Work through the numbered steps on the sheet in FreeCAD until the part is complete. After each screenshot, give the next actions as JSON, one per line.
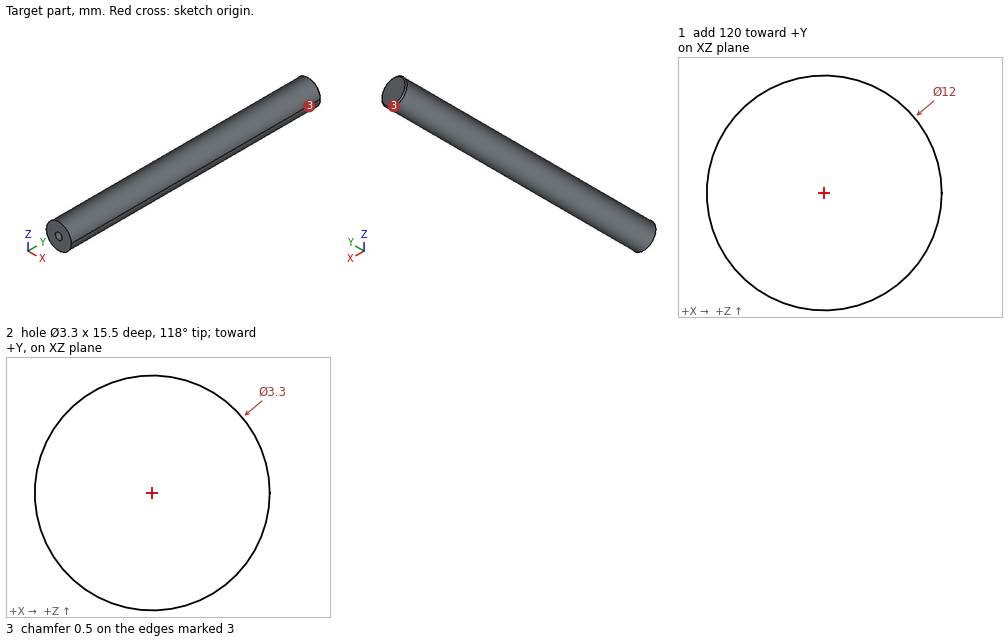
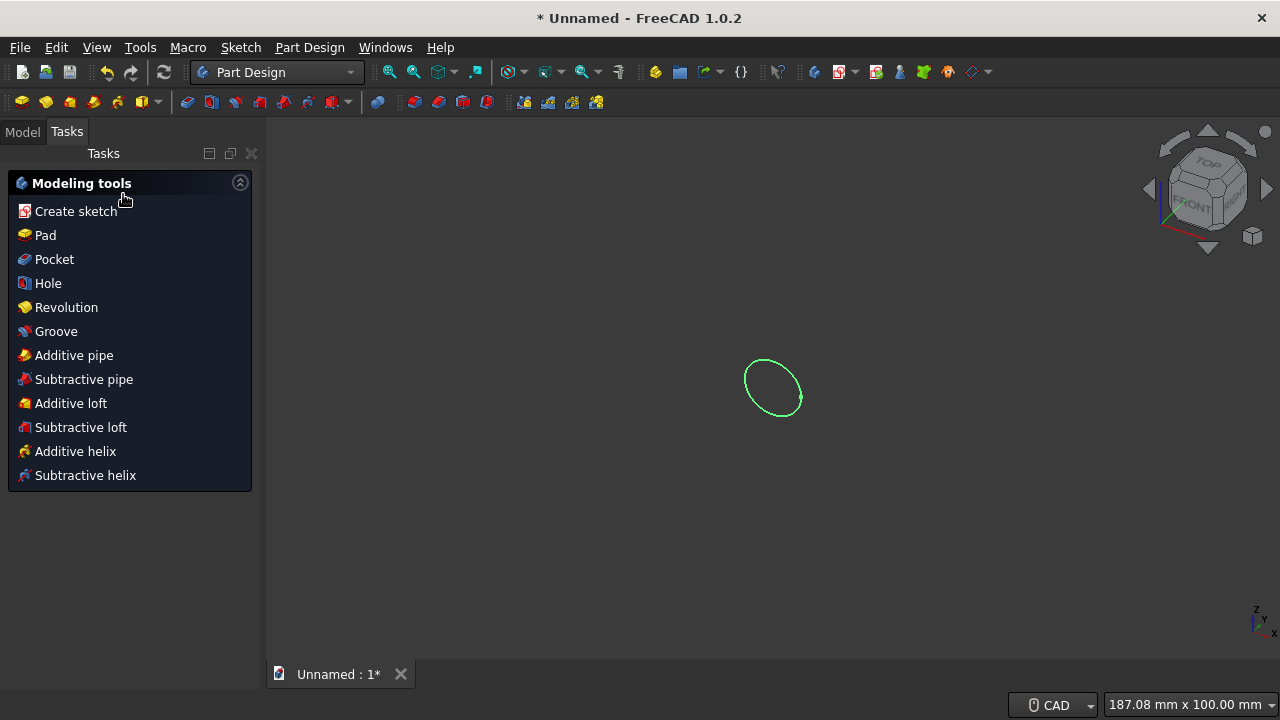
{"action": "left_click", "coordinate": [22, 102]}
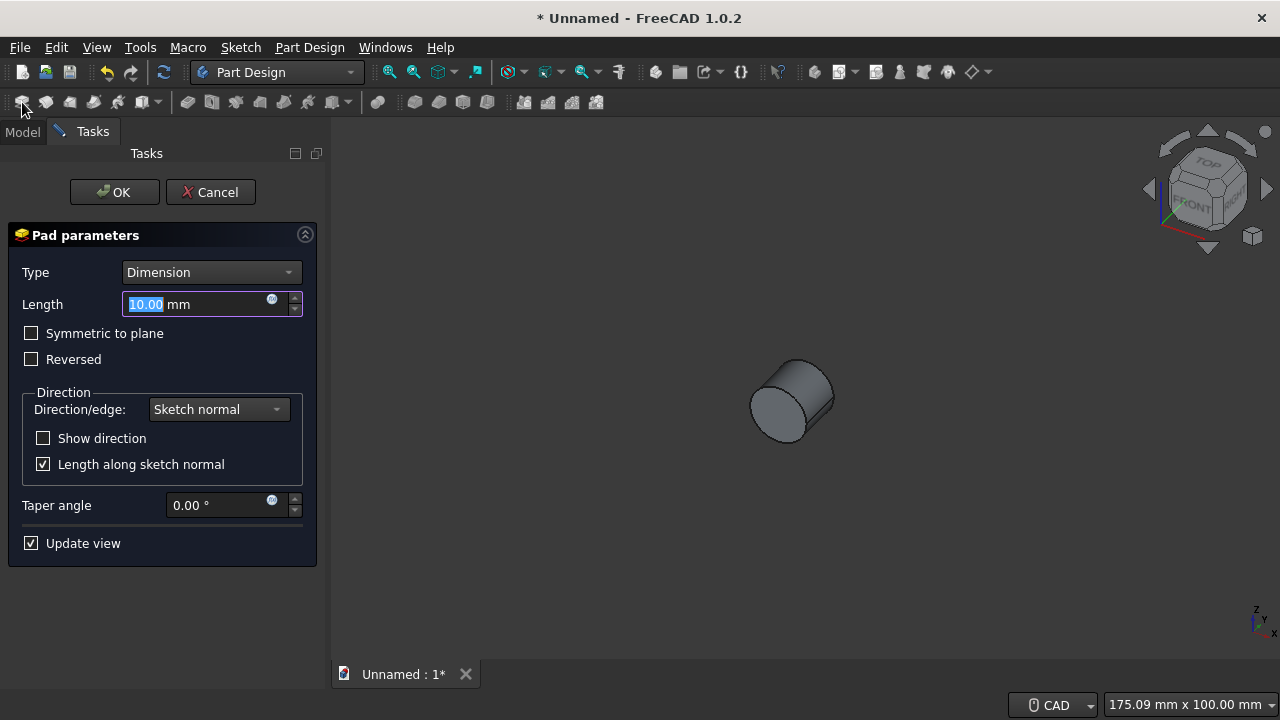
{"action": "type", "text": "120"}
{"action": "key", "text": "Tab"}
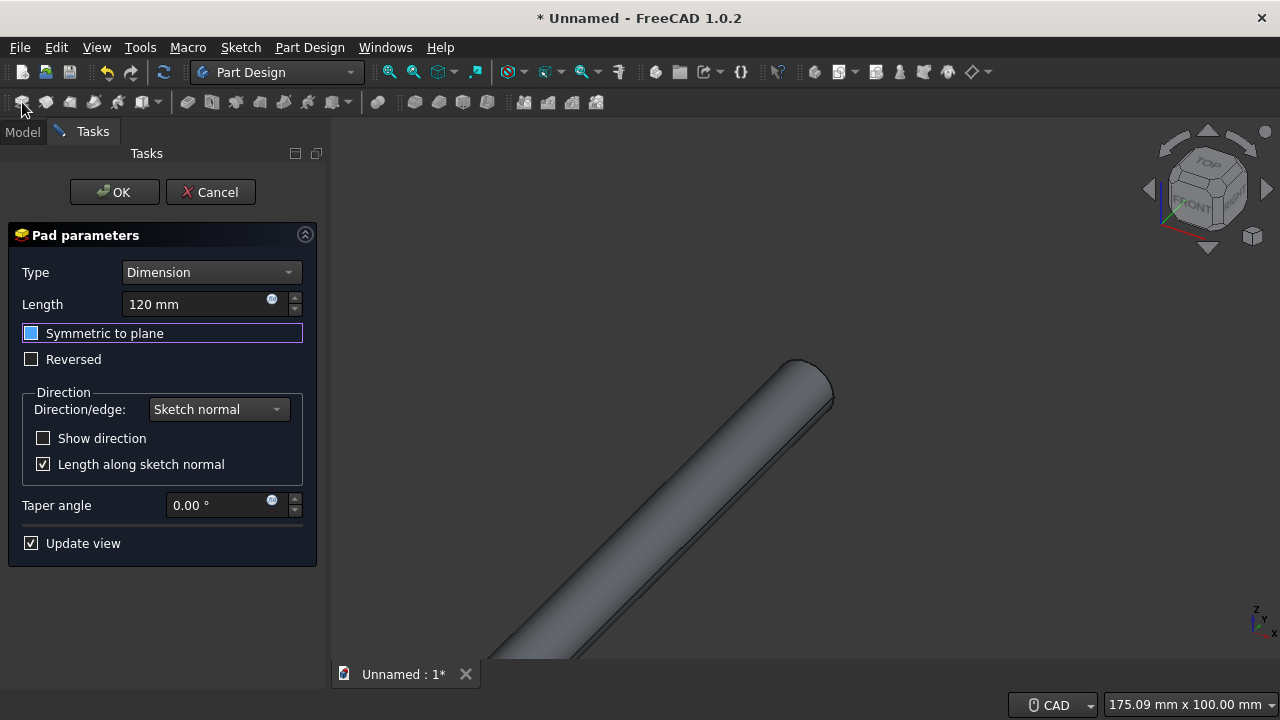
{"action": "left_click", "coordinate": [30, 359]}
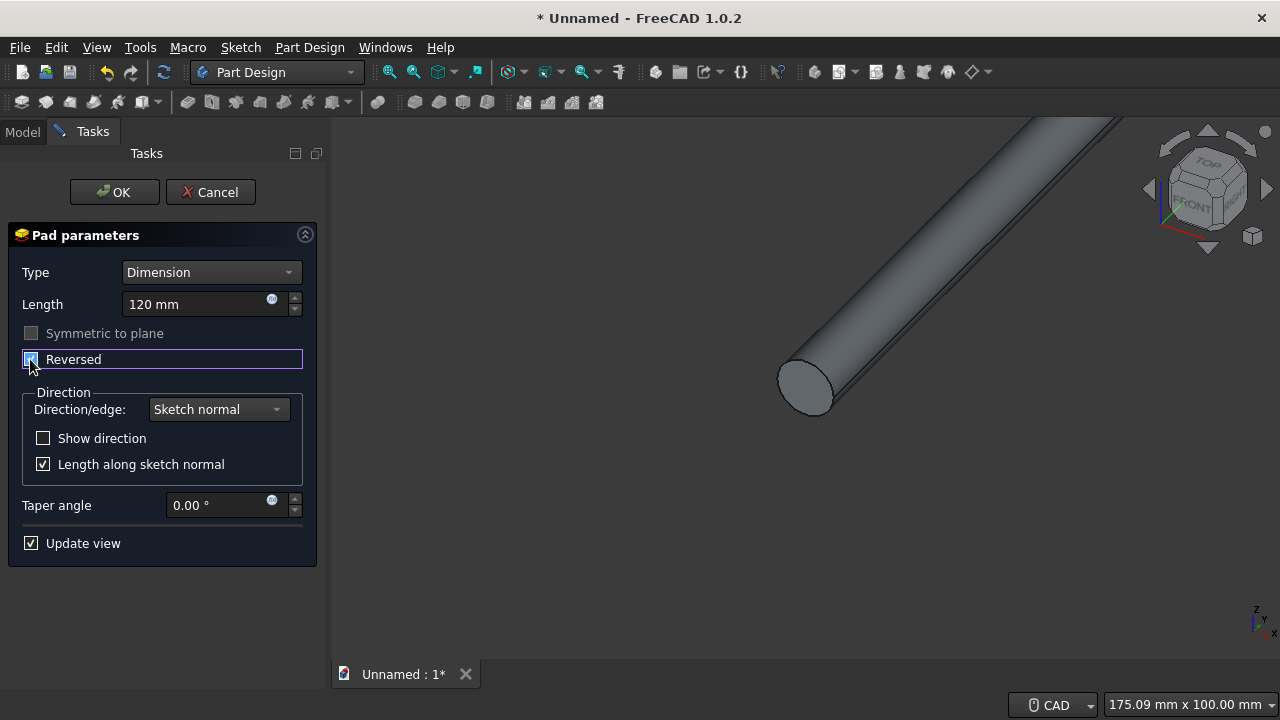
{"action": "left_click", "coordinate": [115, 192]}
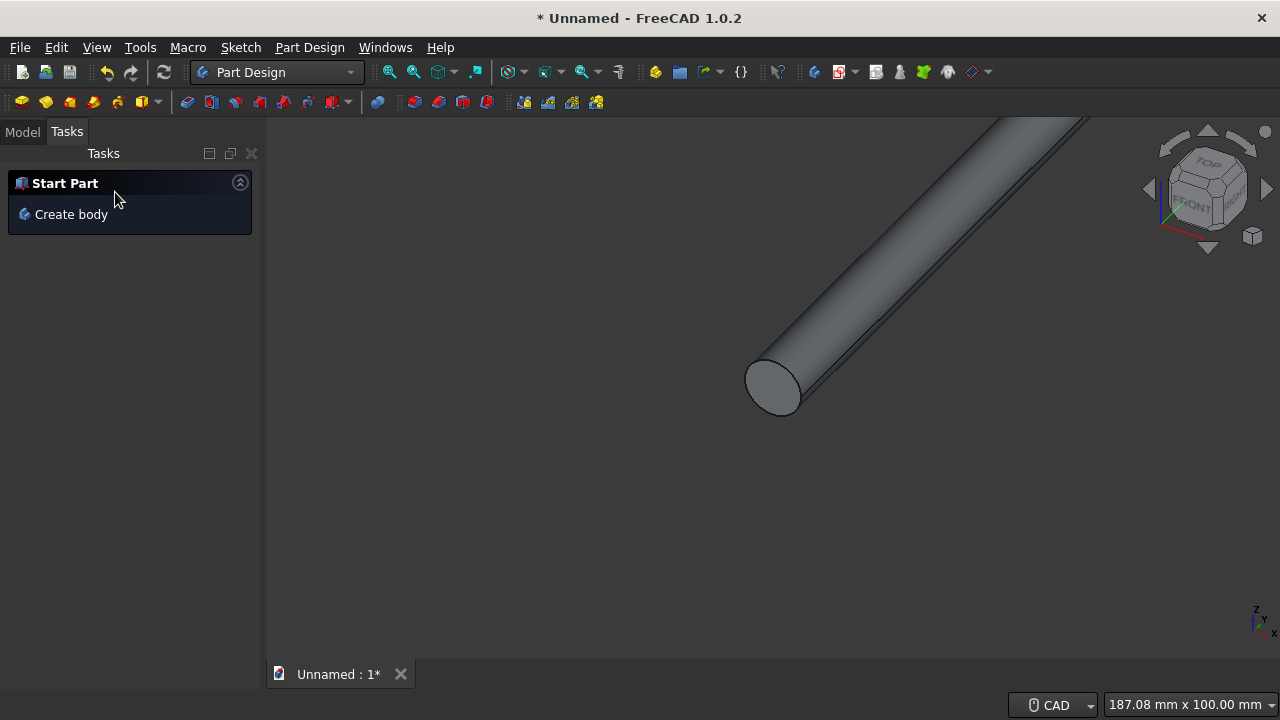
{"action": "left_click", "coordinate": [390, 72]}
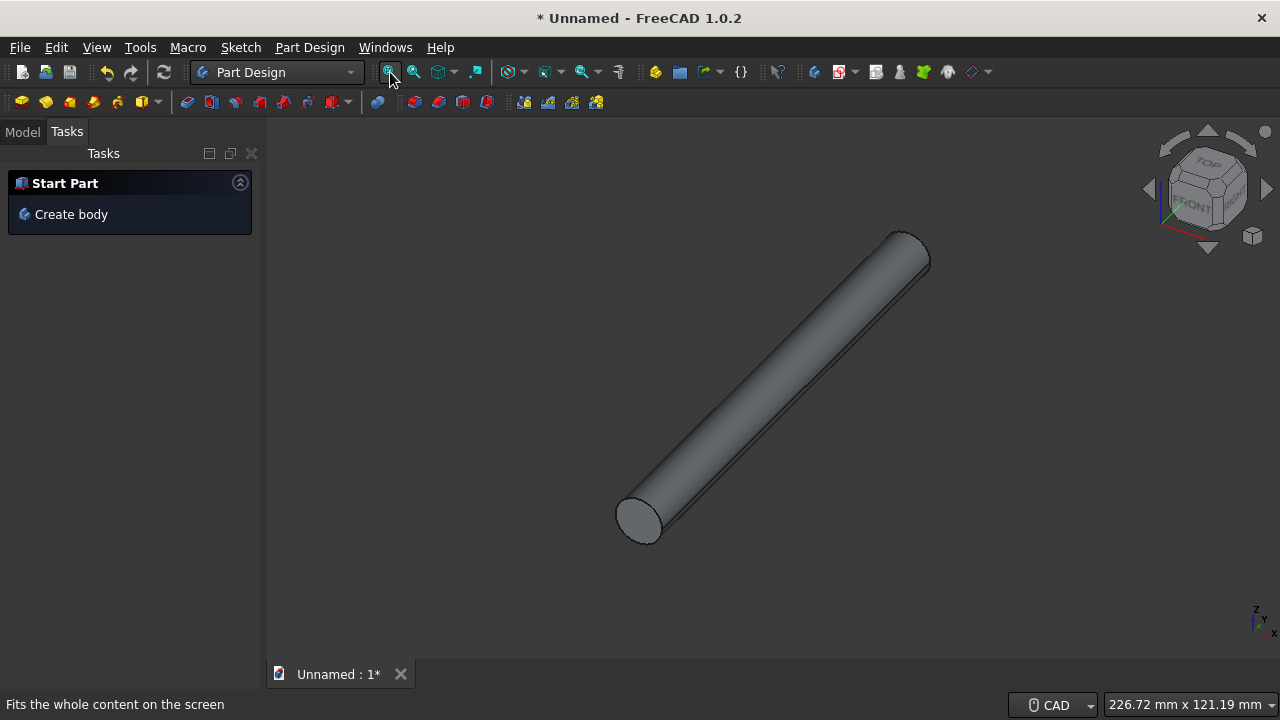
{"action": "left_click", "coordinate": [840, 72]}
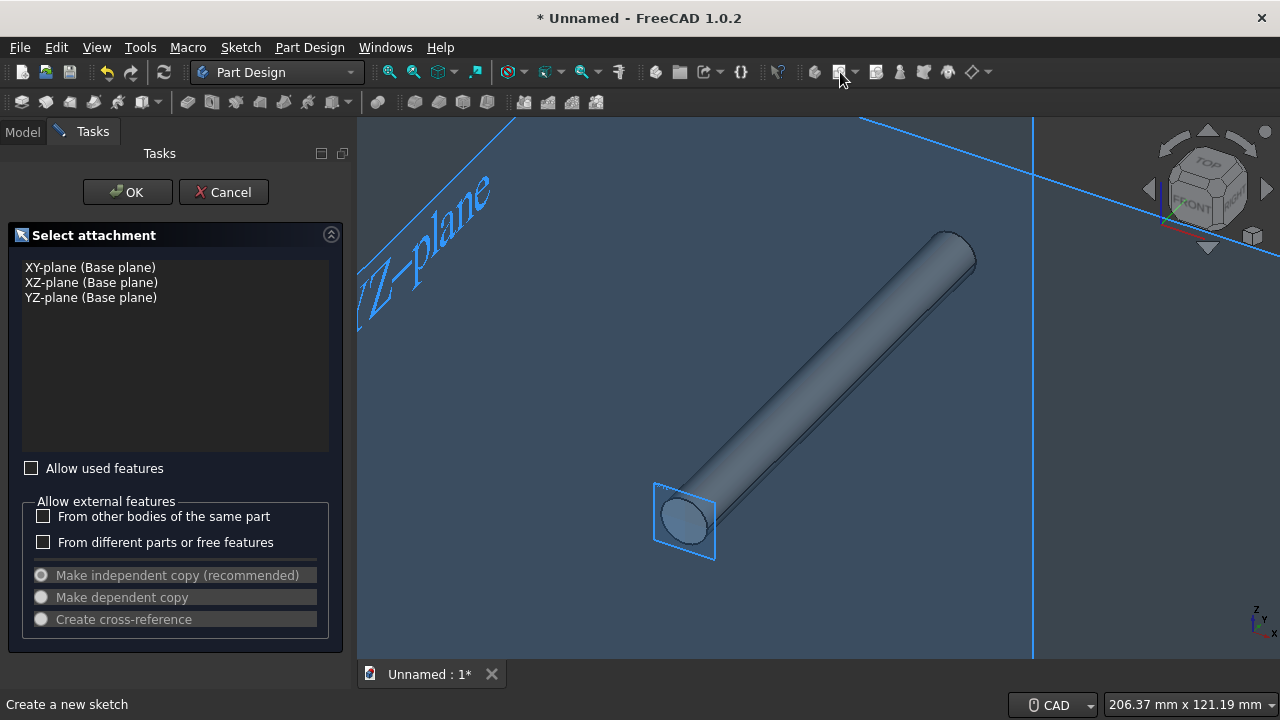
{"action": "left_click", "coordinate": [82, 282]}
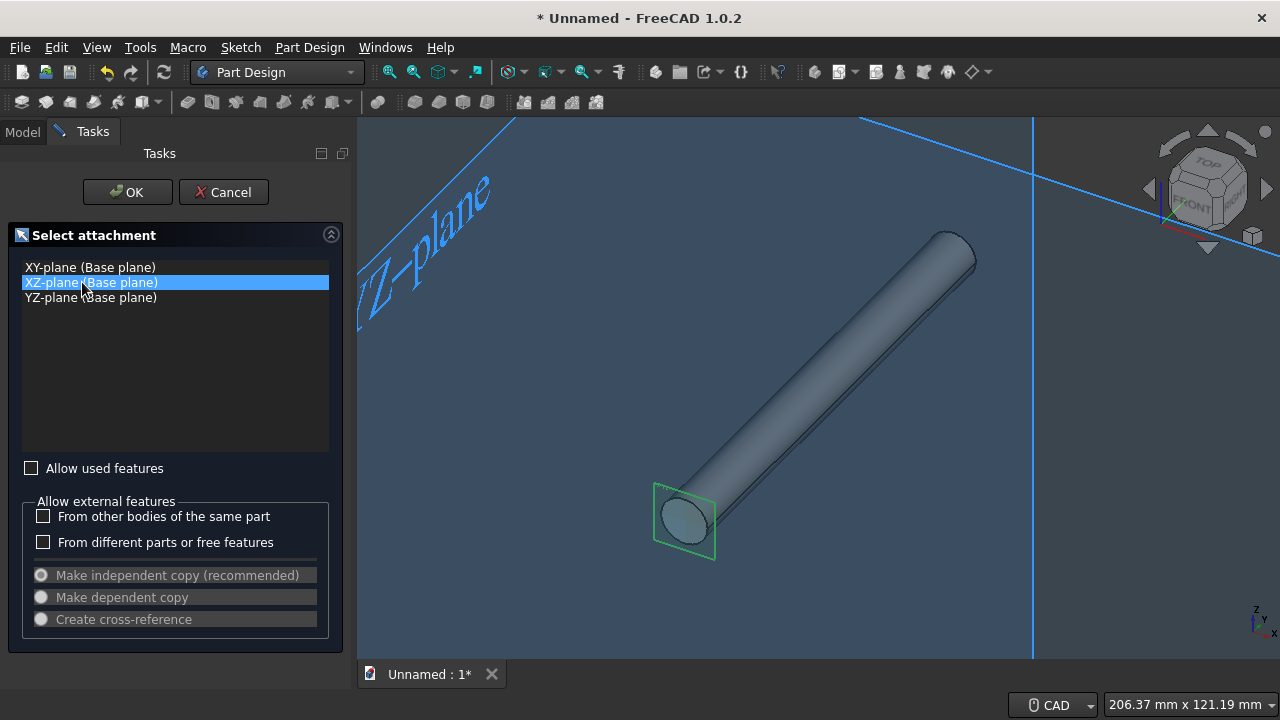
{"action": "left_click", "coordinate": [128, 192]}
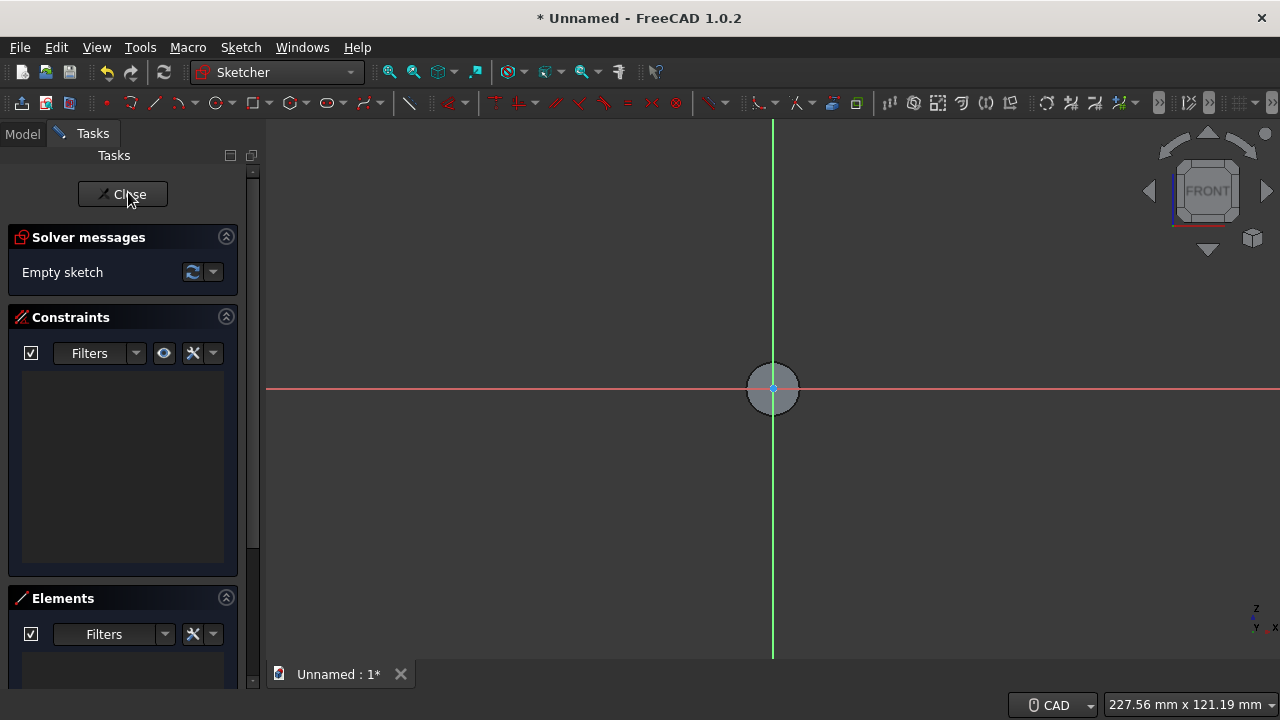
{"action": "scroll", "coordinate": [777, 389], "scroll_direction": "up", "scroll_amount": 15}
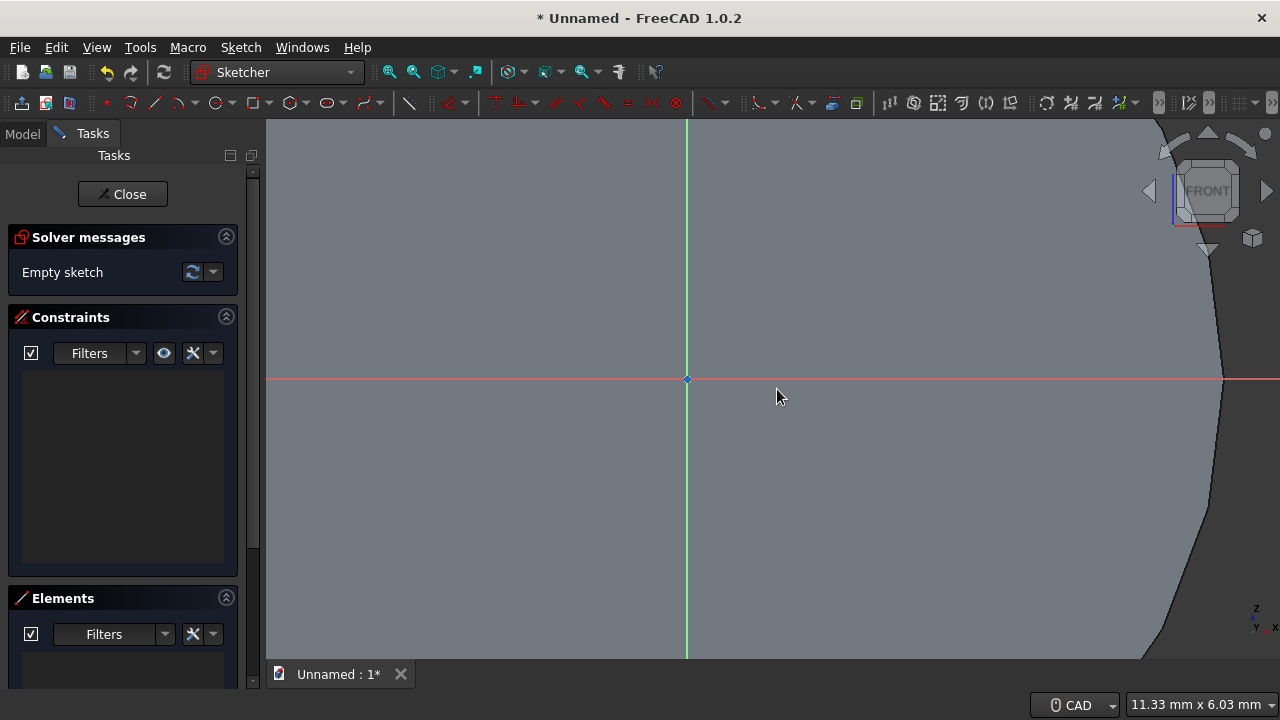
{"action": "left_click", "coordinate": [216, 104]}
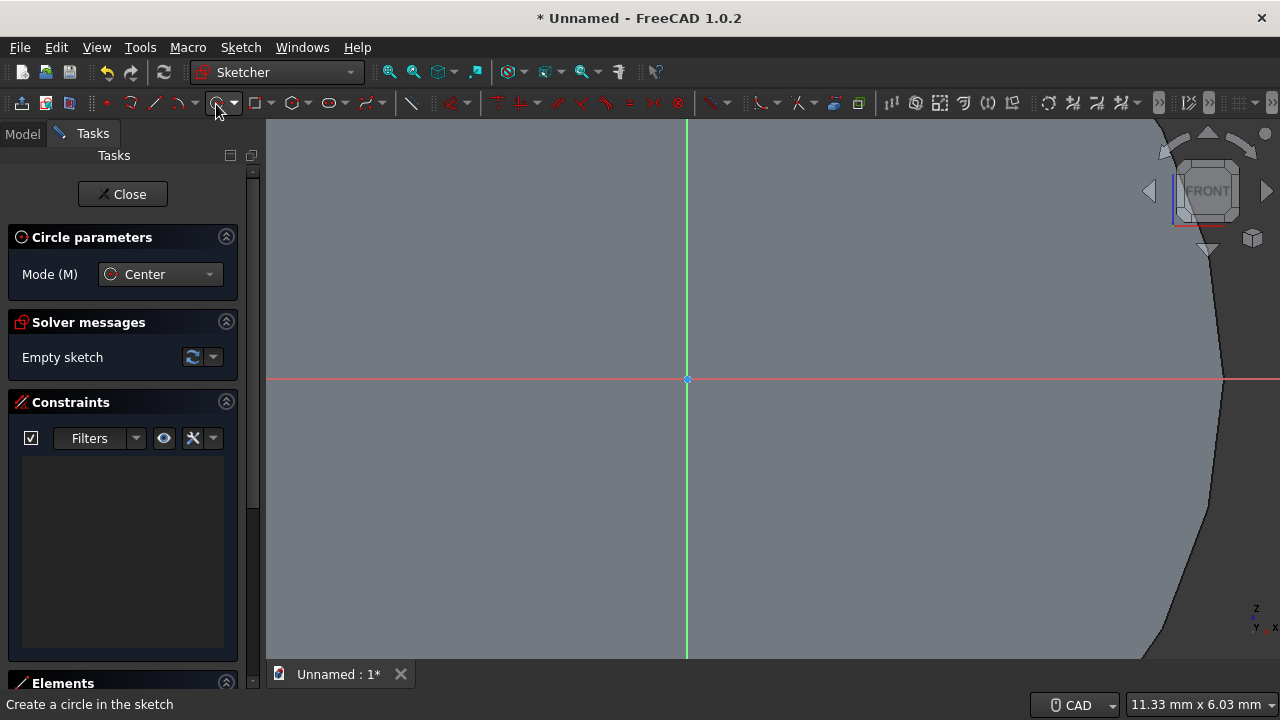
{"action": "left_click", "coordinate": [687, 379]}
{"action": "left_click", "coordinate": [791, 275]}
{"action": "key", "text": "Escape"}